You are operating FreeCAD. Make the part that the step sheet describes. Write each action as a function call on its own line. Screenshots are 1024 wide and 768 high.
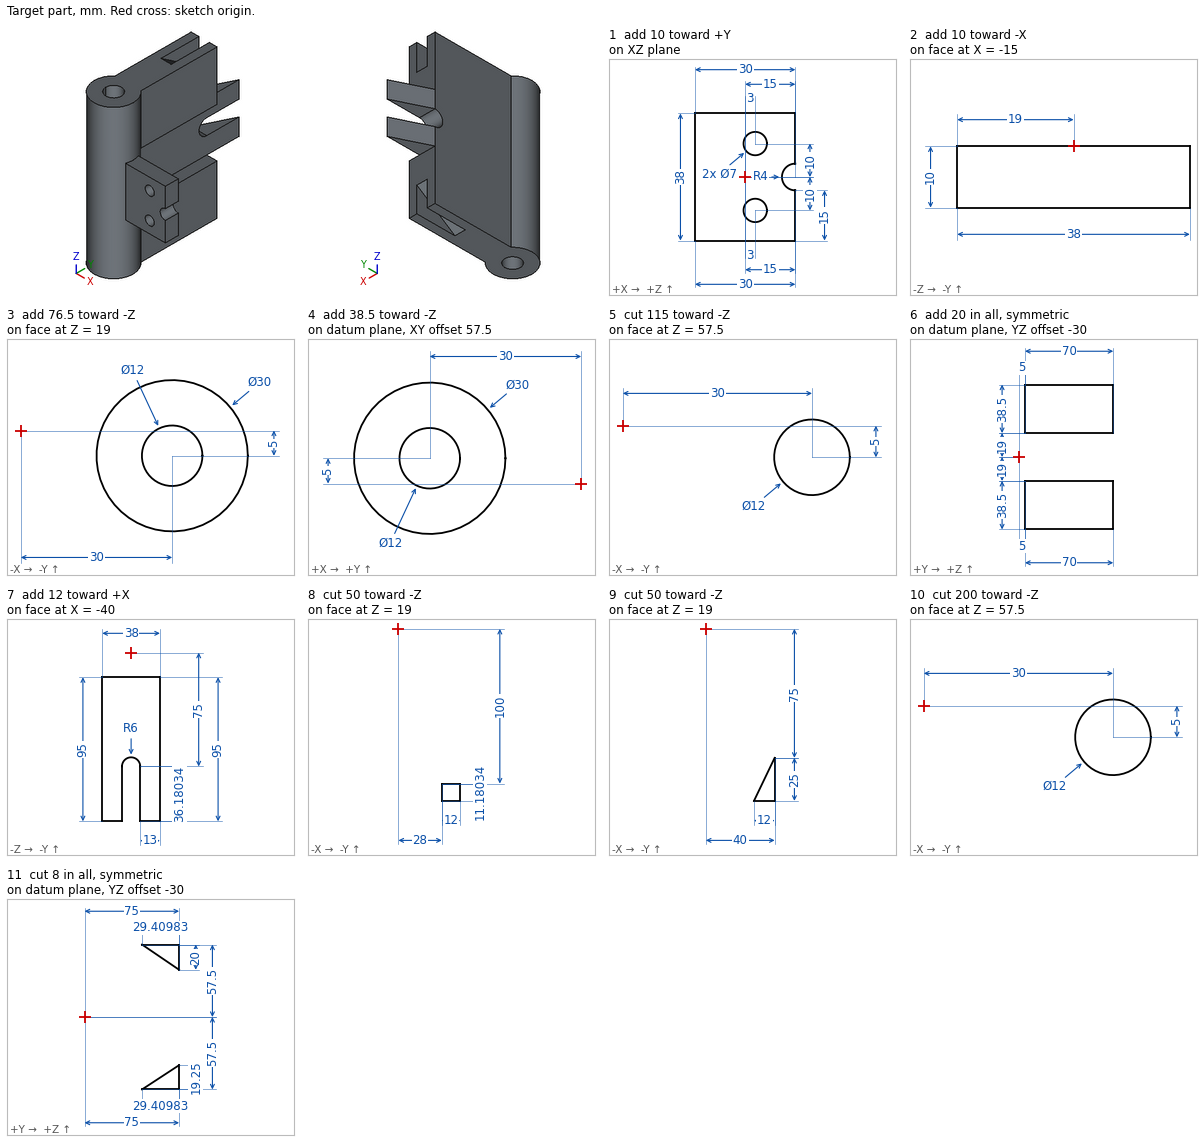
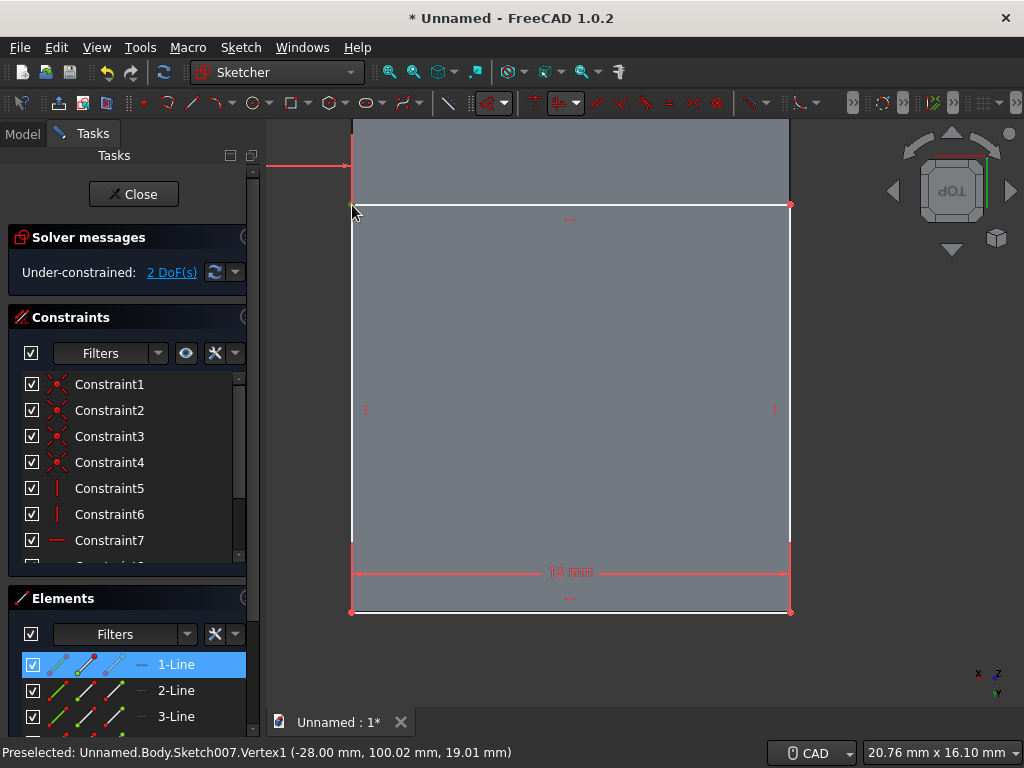
click(506, 104)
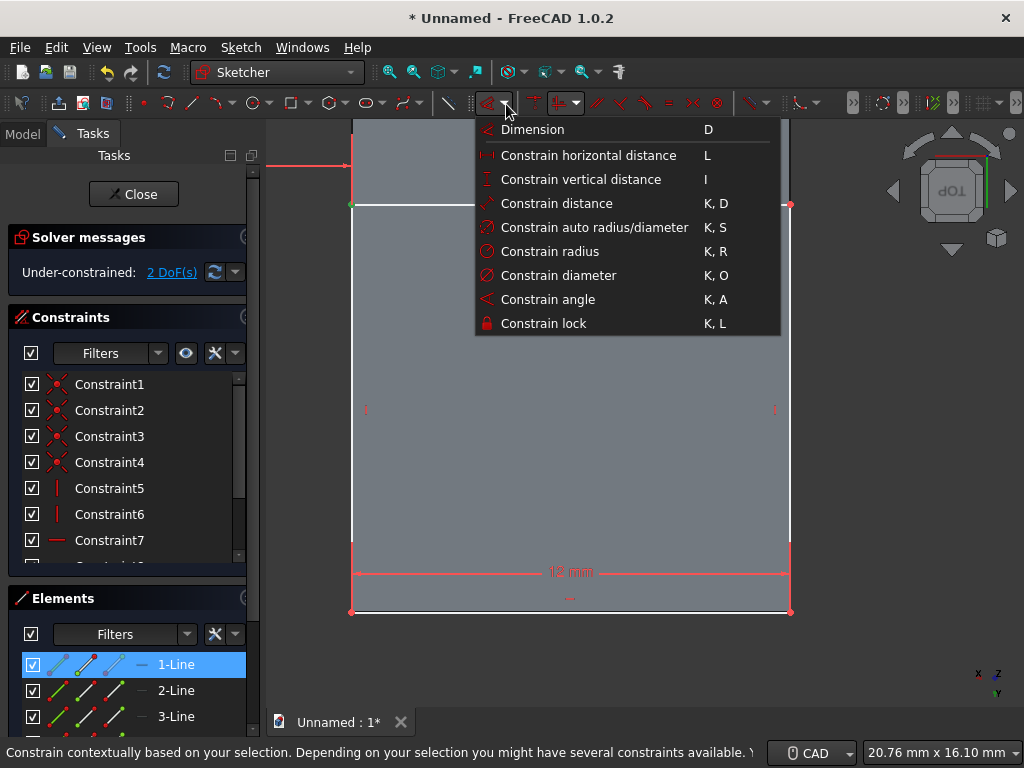
click(628, 179)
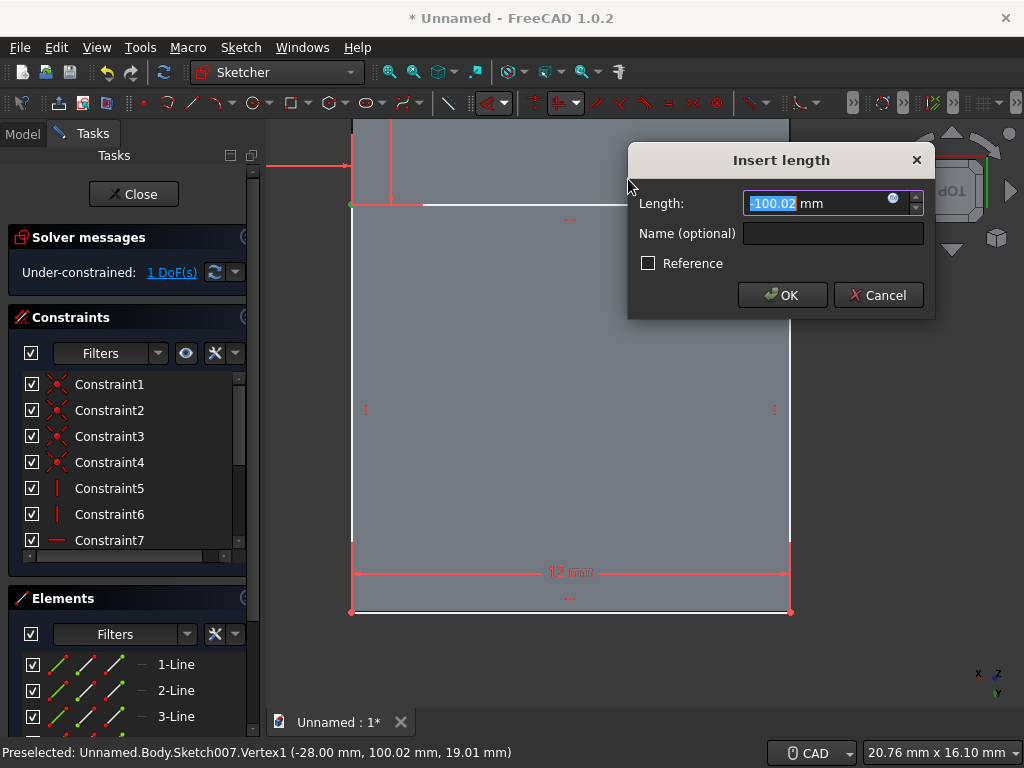
text(-100)
key(Return)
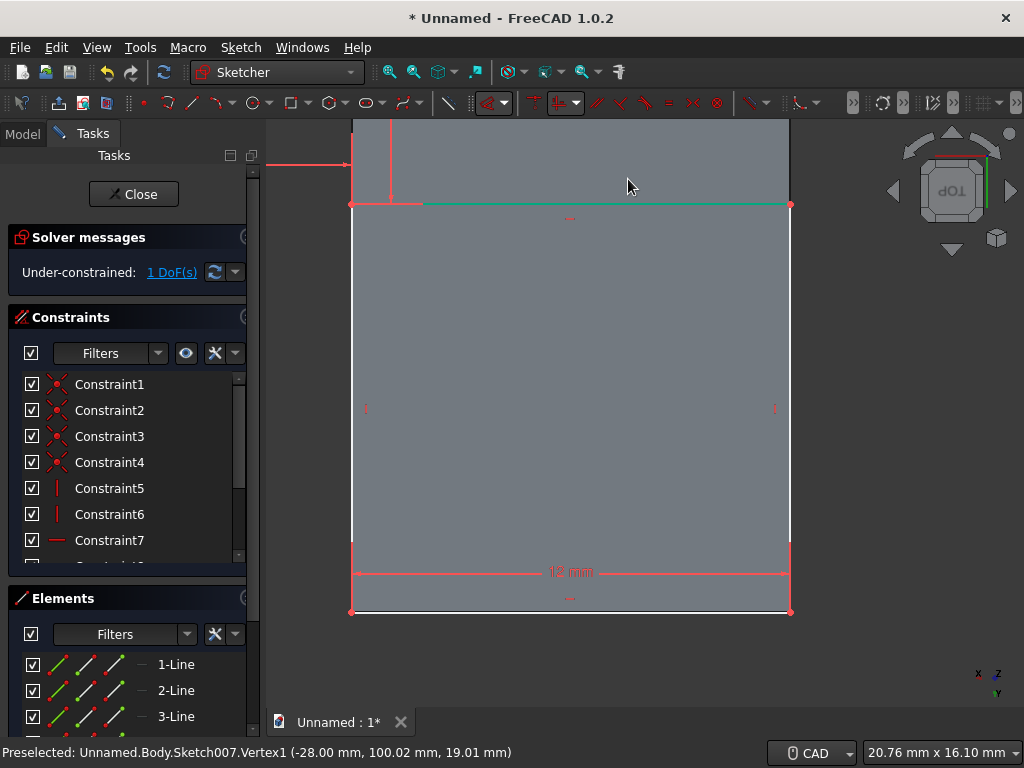
click(352, 327)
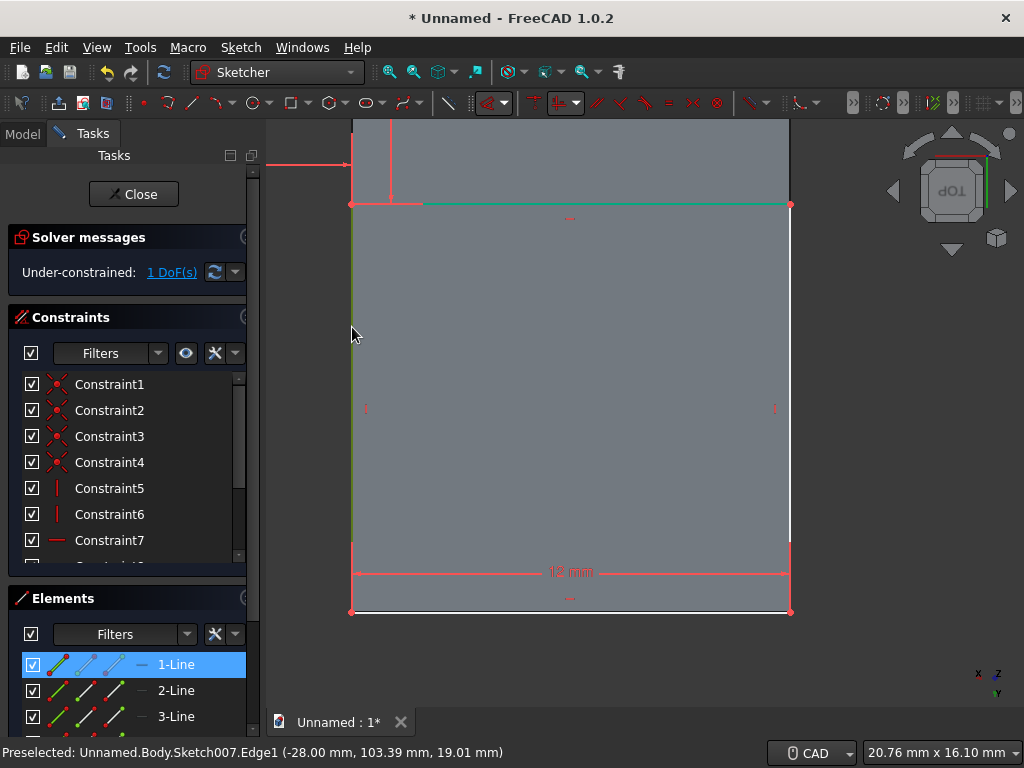
key(i)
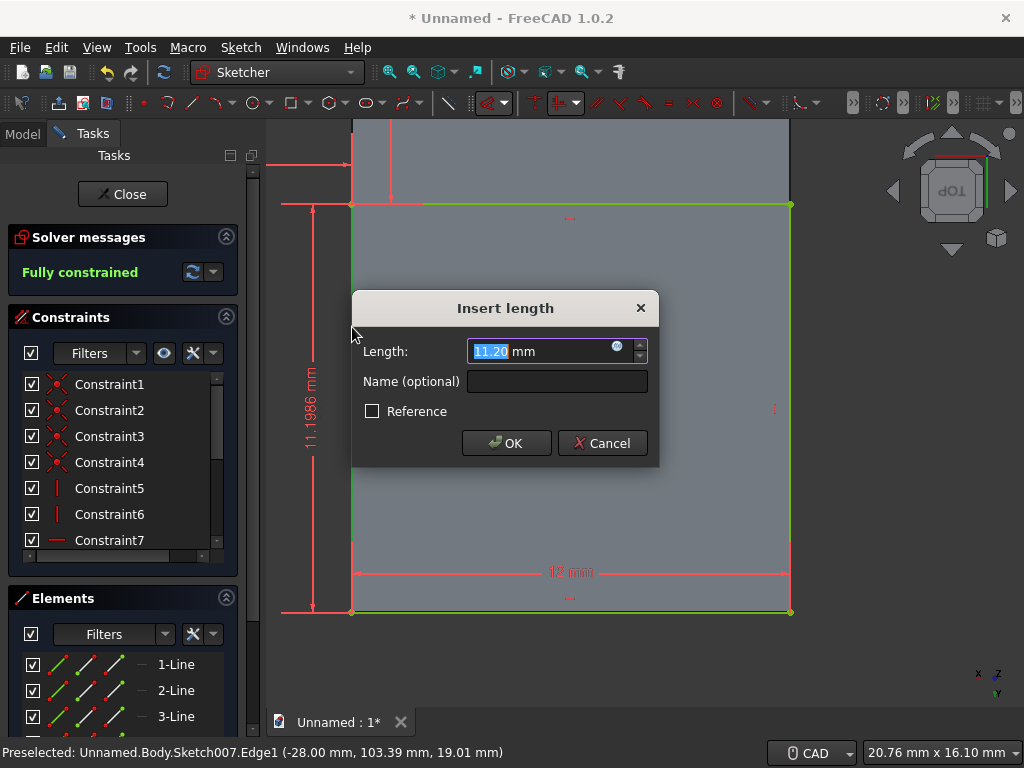
text(11.18034)
key(Return)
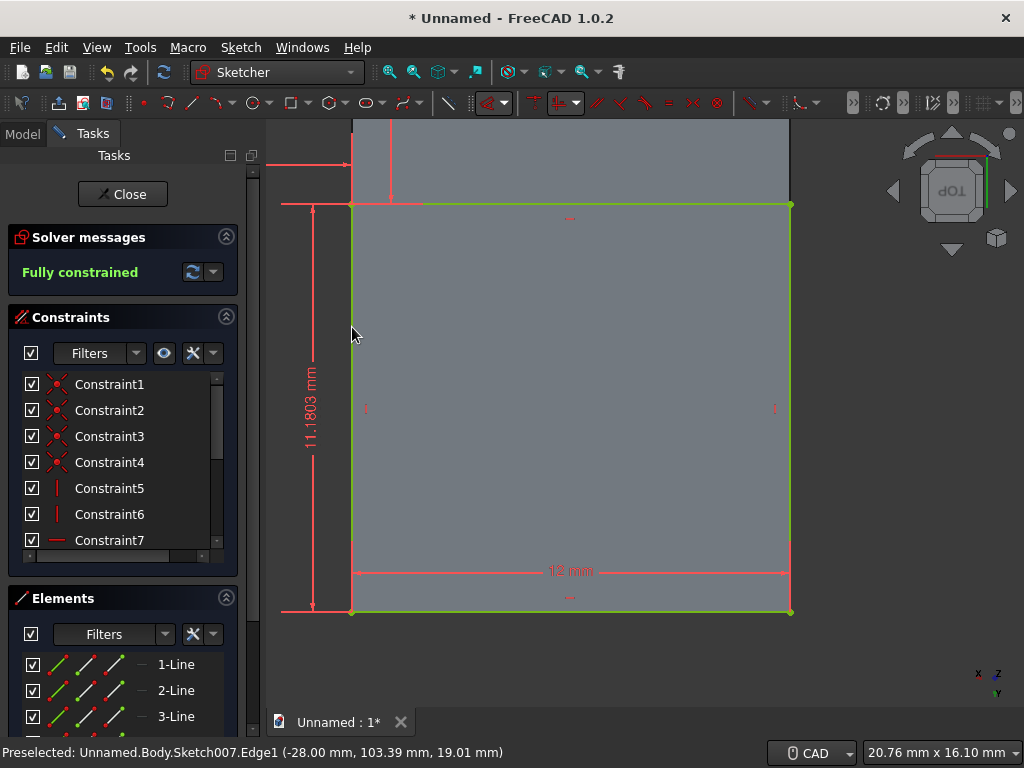
click(123, 194)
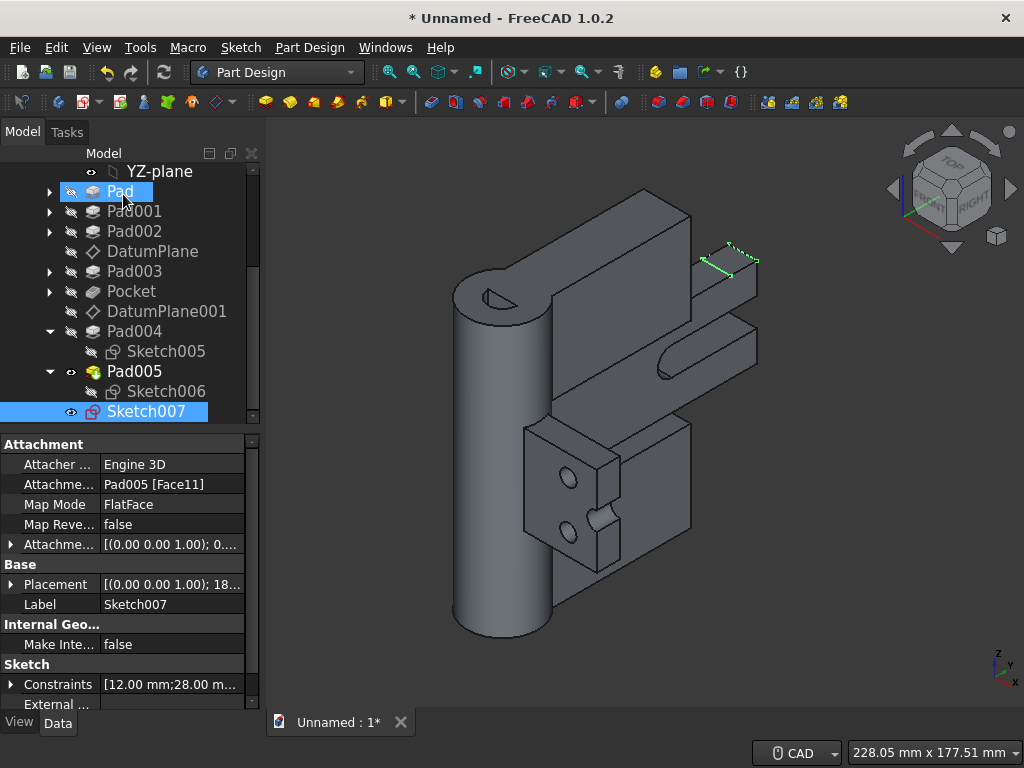
click(432, 102)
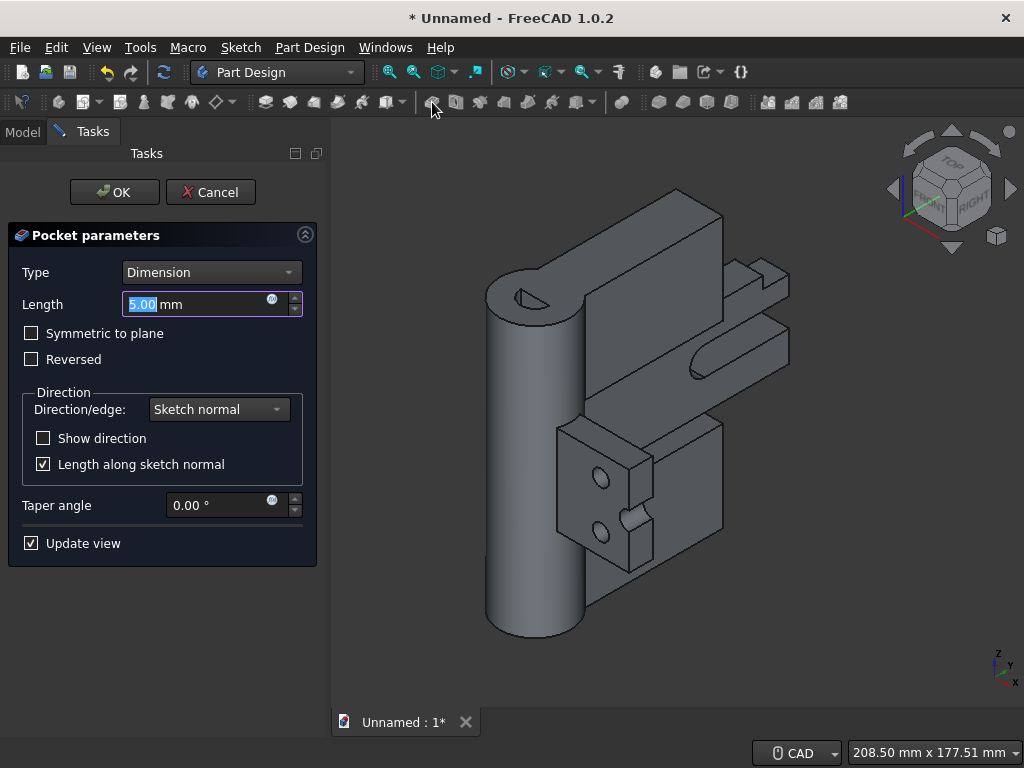
text(50)
key(Tab)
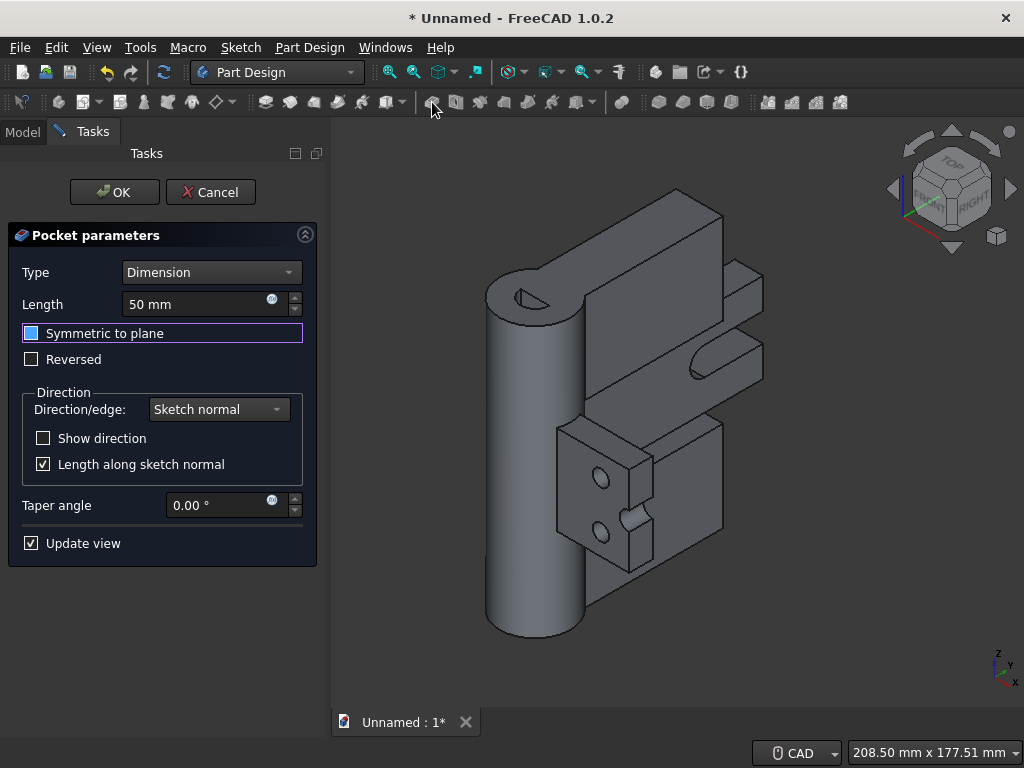
click(115, 192)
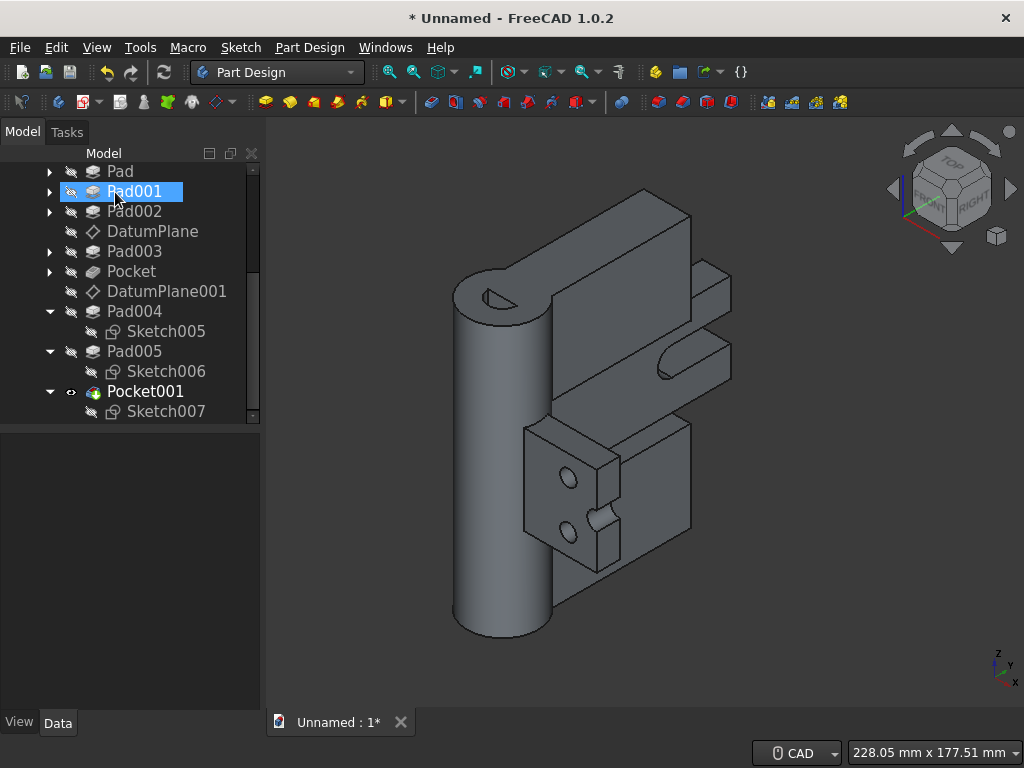
click(593, 453)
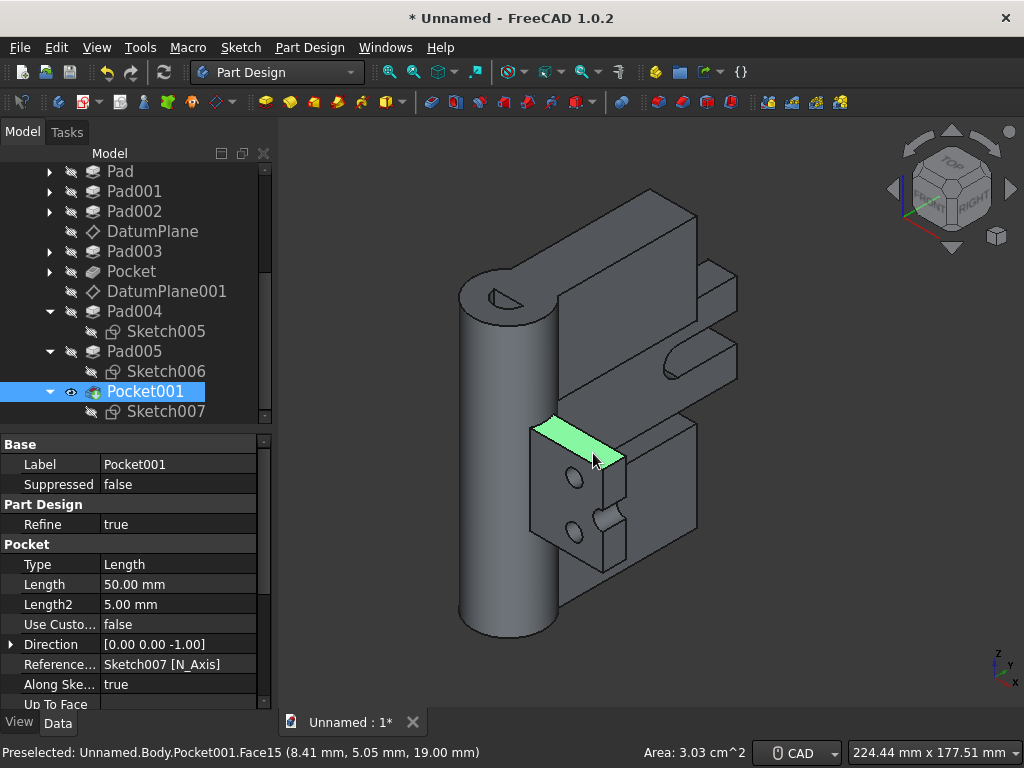
click(84, 102)